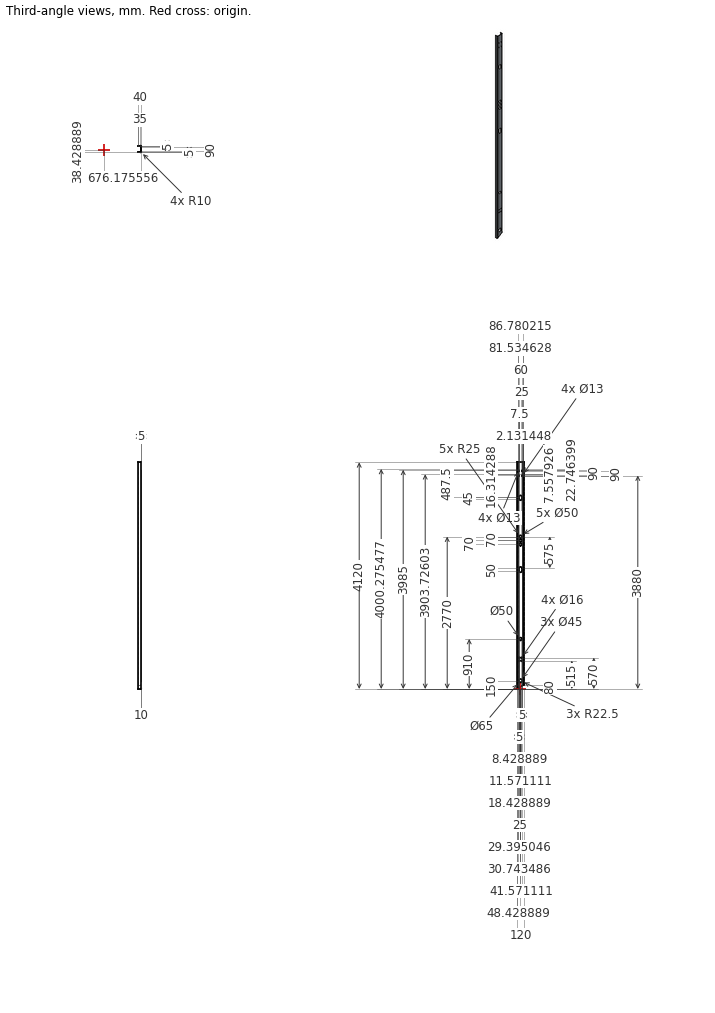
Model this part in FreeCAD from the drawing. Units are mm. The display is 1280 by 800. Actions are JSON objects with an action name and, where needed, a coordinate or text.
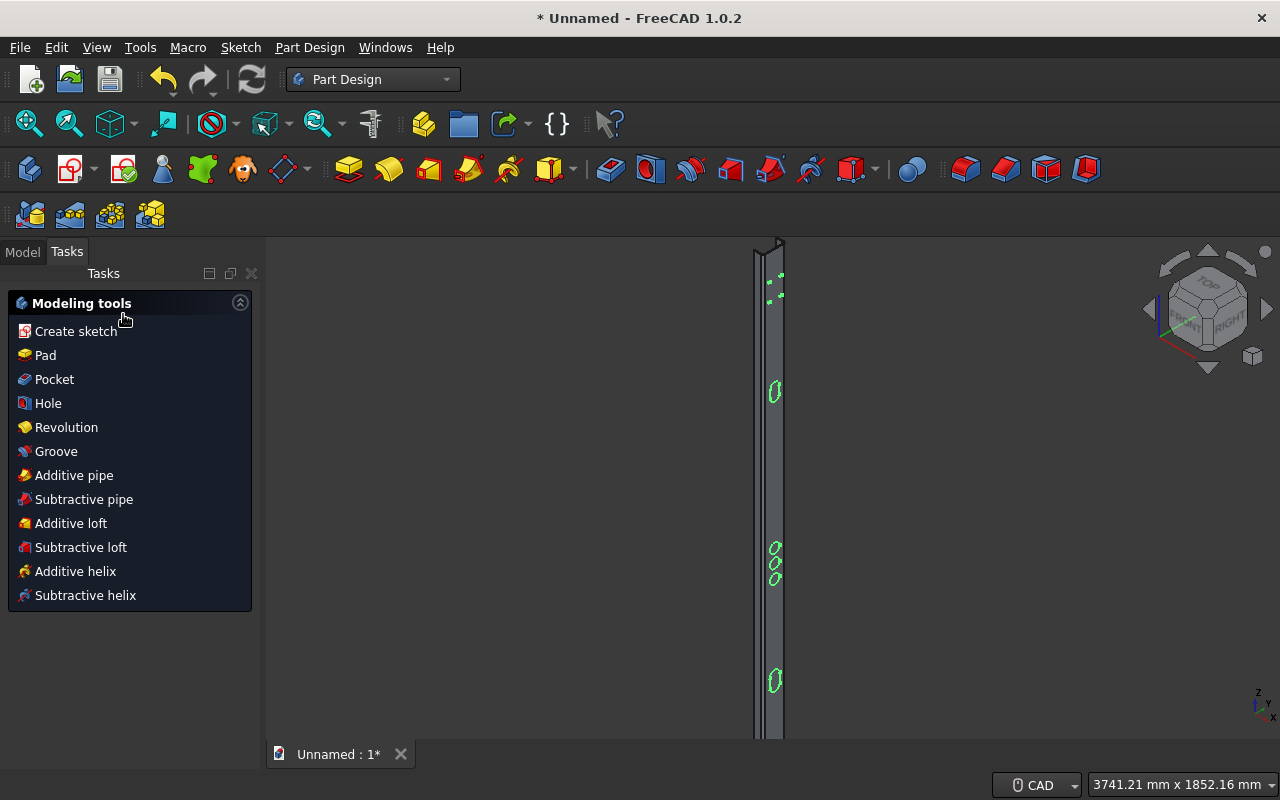
{"action": "left_click", "coordinate": [612, 170]}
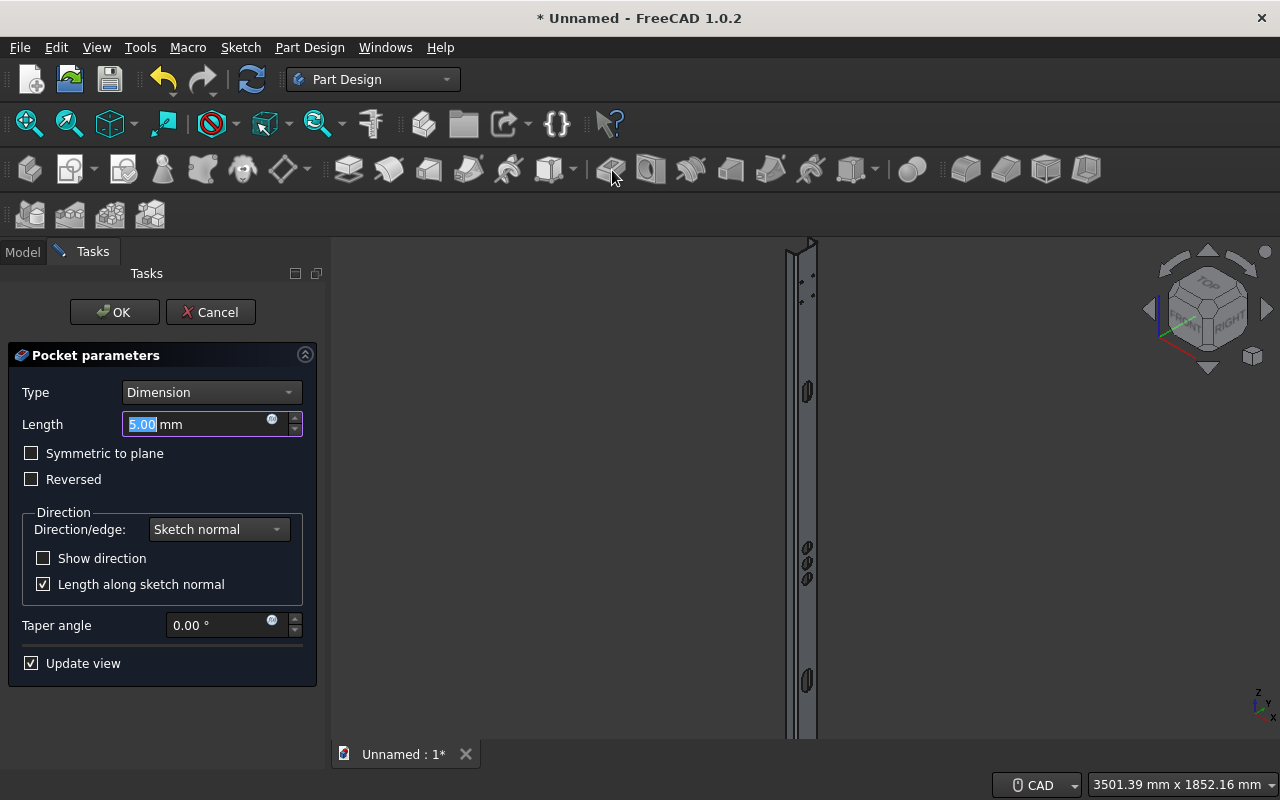
{"action": "type", "text": "10"}
{"action": "key", "text": "Tab"}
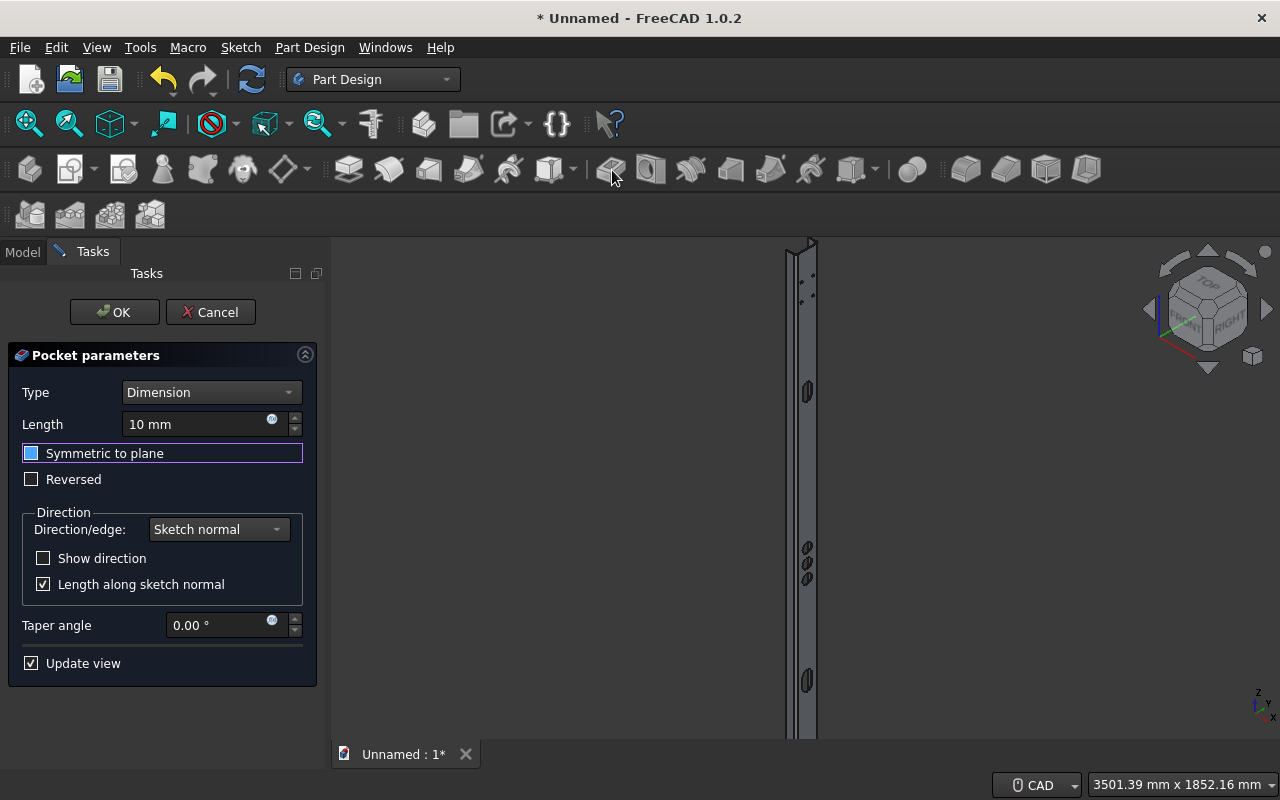
{"action": "left_click", "coordinate": [115, 312]}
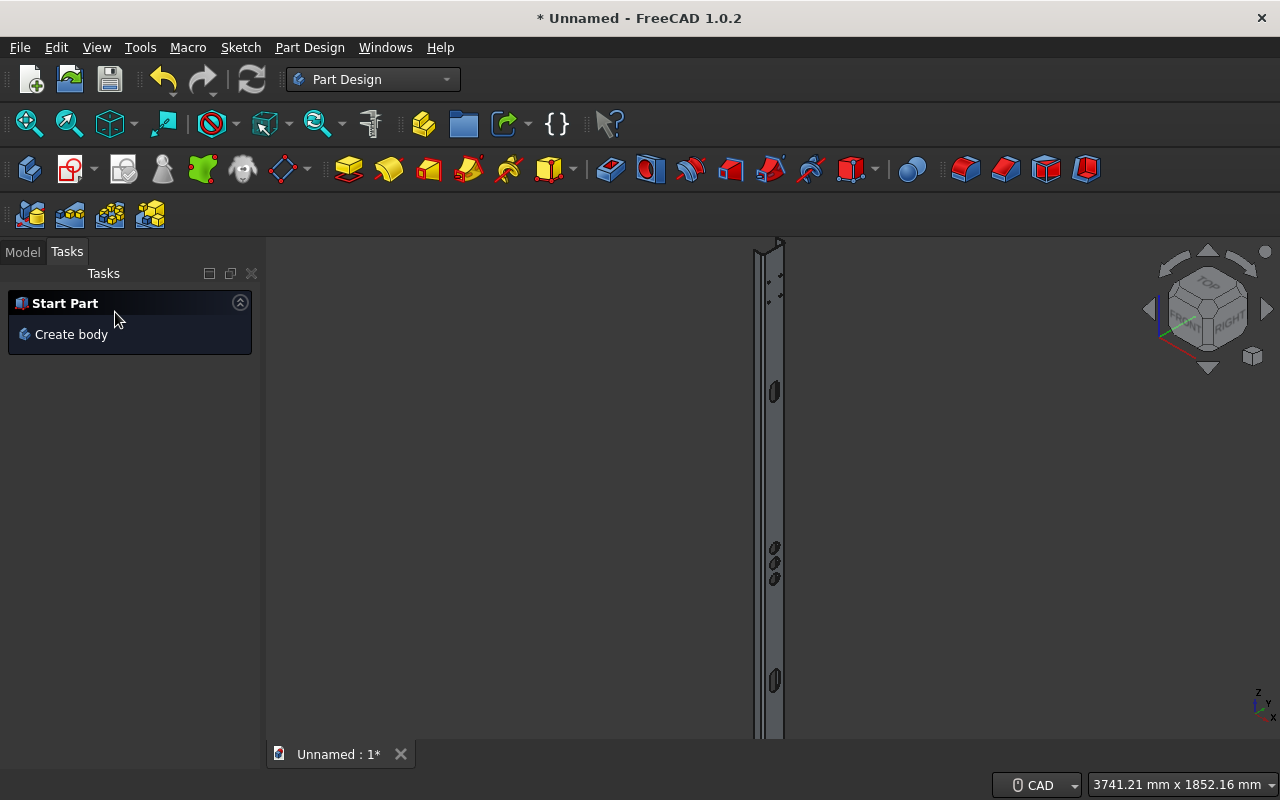
{"action": "left_click", "coordinate": [30, 124]}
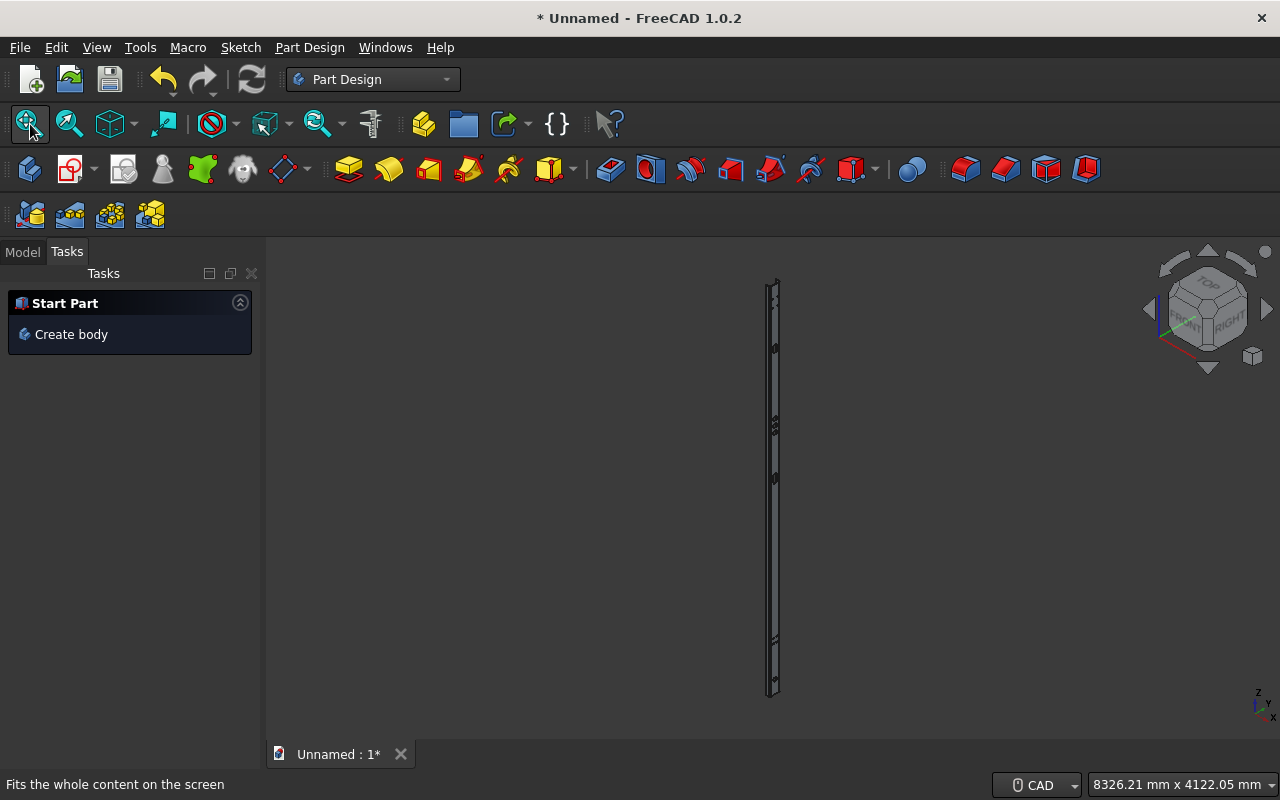
{"action": "scroll", "coordinate": [775, 313], "scroll_direction": "up", "scroll_amount": 4}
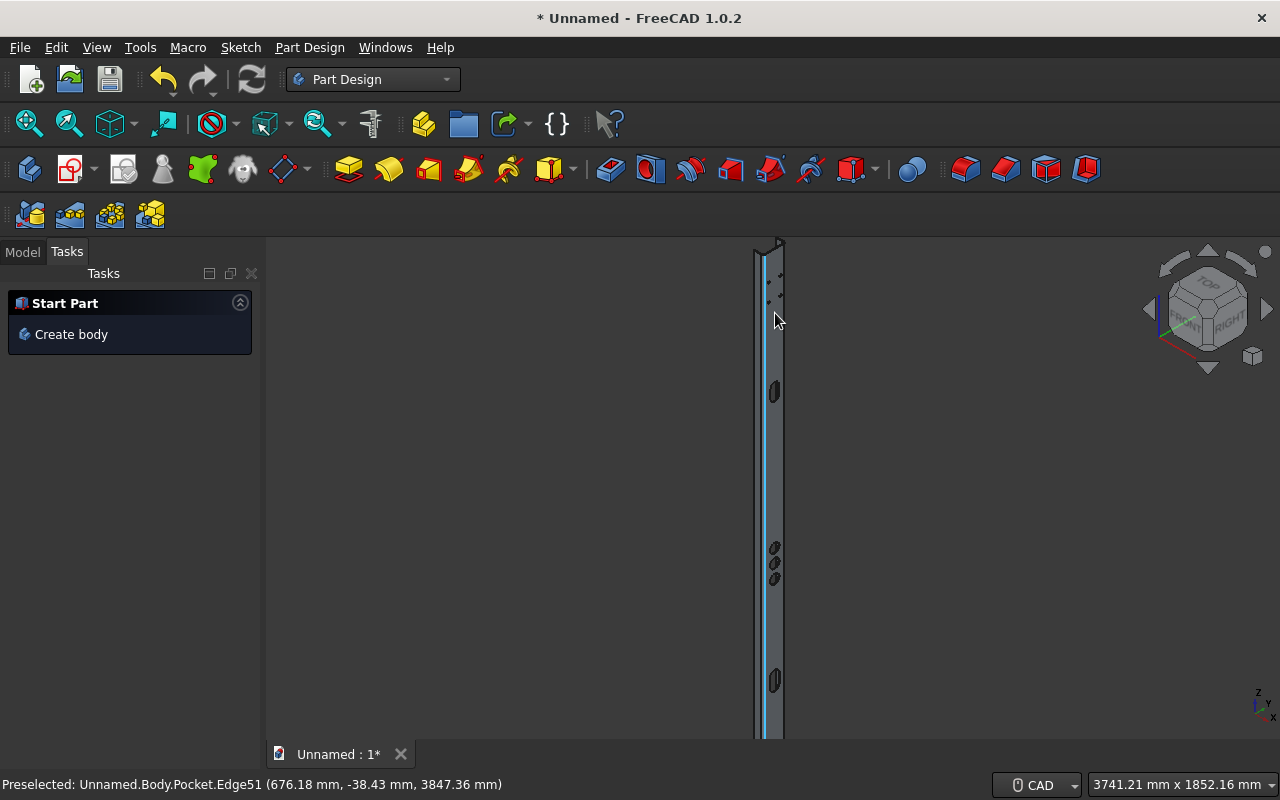
{"action": "left_click", "coordinate": [775, 313]}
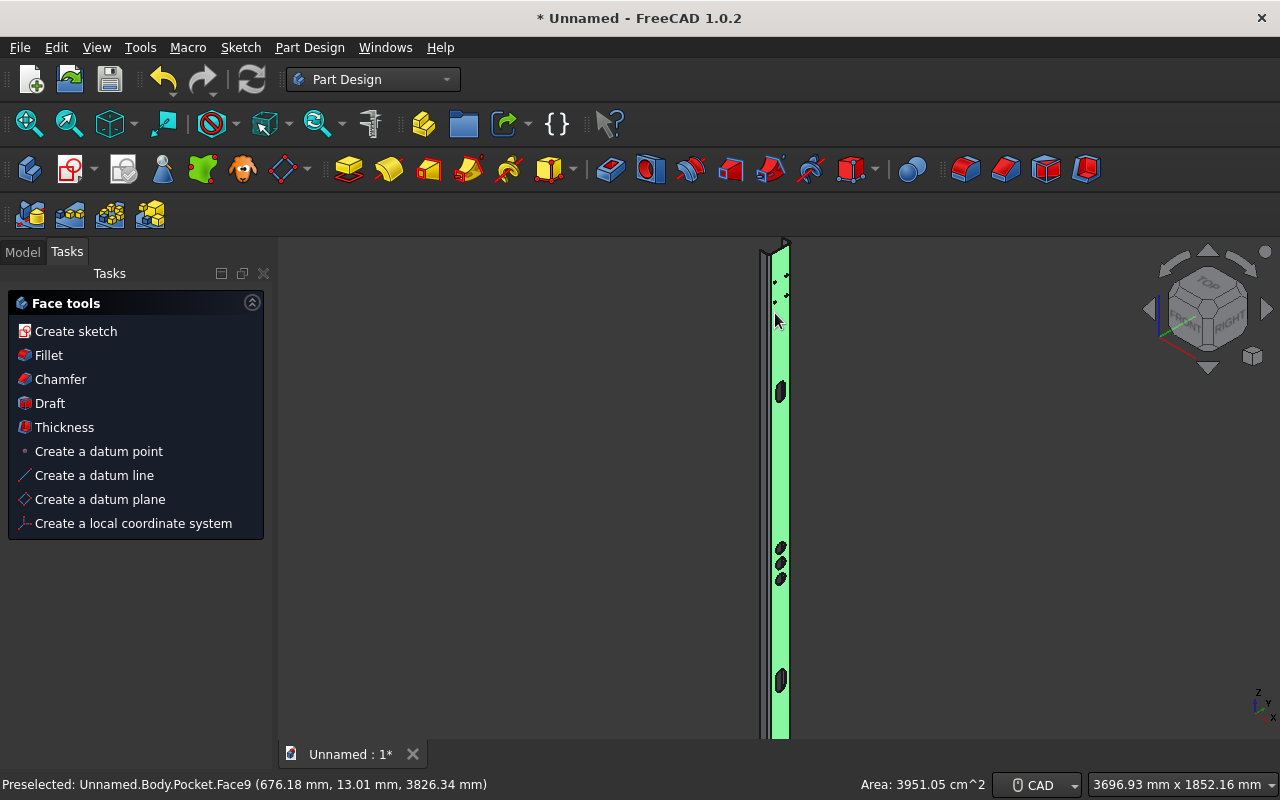
{"action": "left_click", "coordinate": [70, 170]}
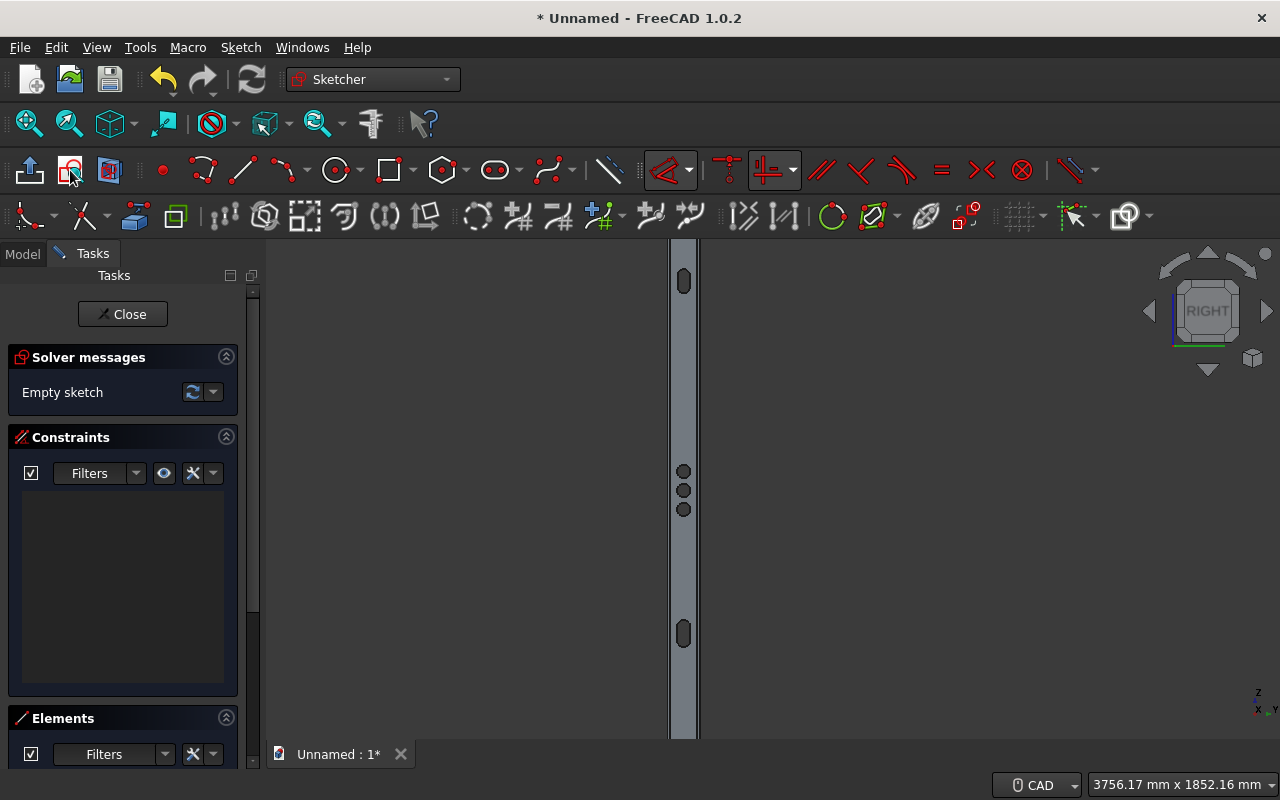
{"action": "scroll", "coordinate": [704, 489], "scroll_direction": "down", "scroll_amount": 5}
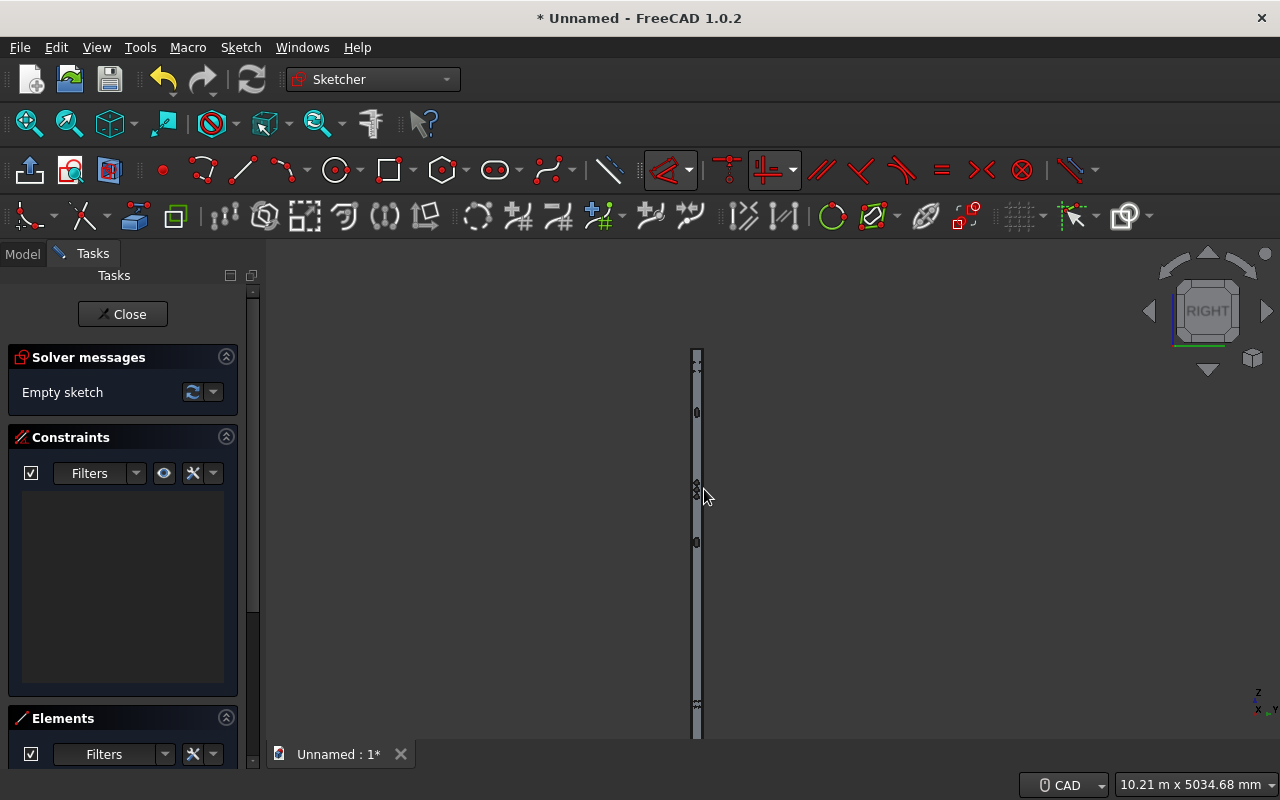
{"action": "scroll", "coordinate": [696, 677], "scroll_direction": "up", "scroll_amount": 15}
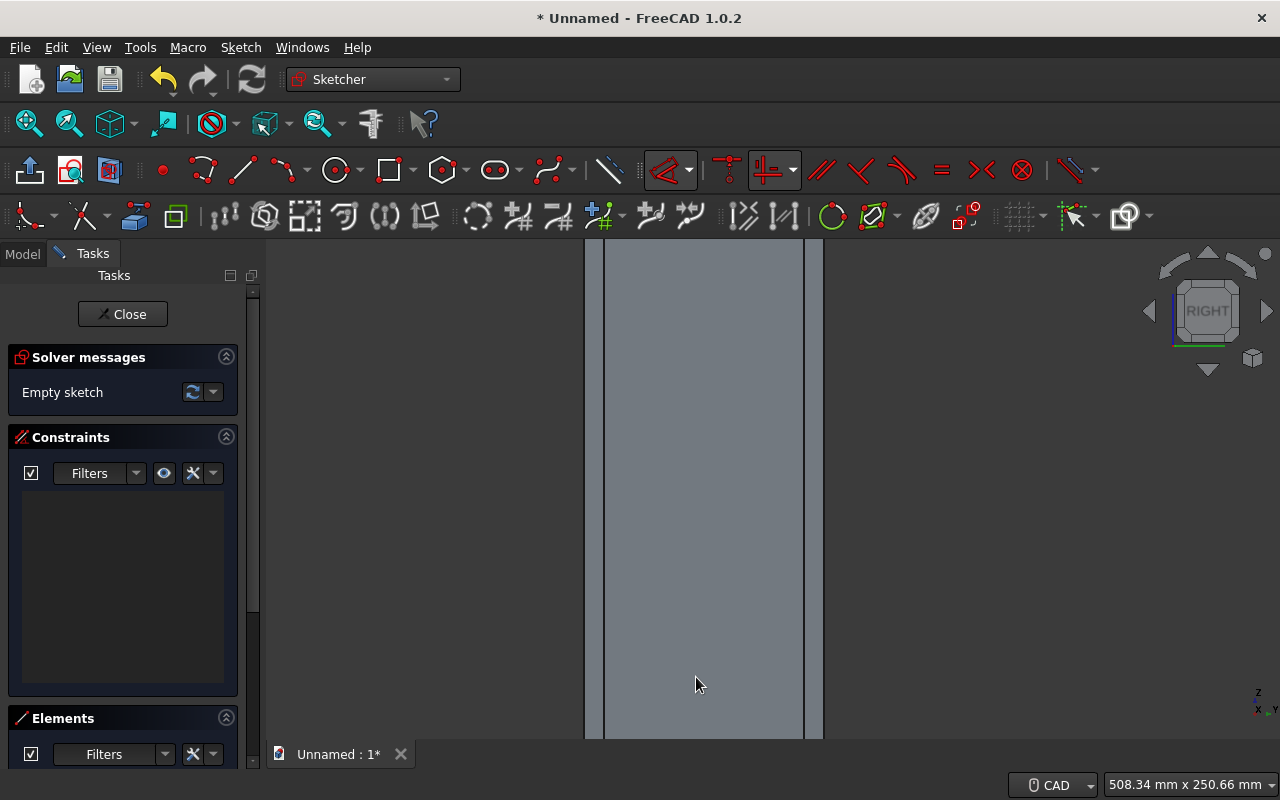
{"action": "scroll", "coordinate": [704, 465], "scroll_direction": "up", "scroll_amount": 6}